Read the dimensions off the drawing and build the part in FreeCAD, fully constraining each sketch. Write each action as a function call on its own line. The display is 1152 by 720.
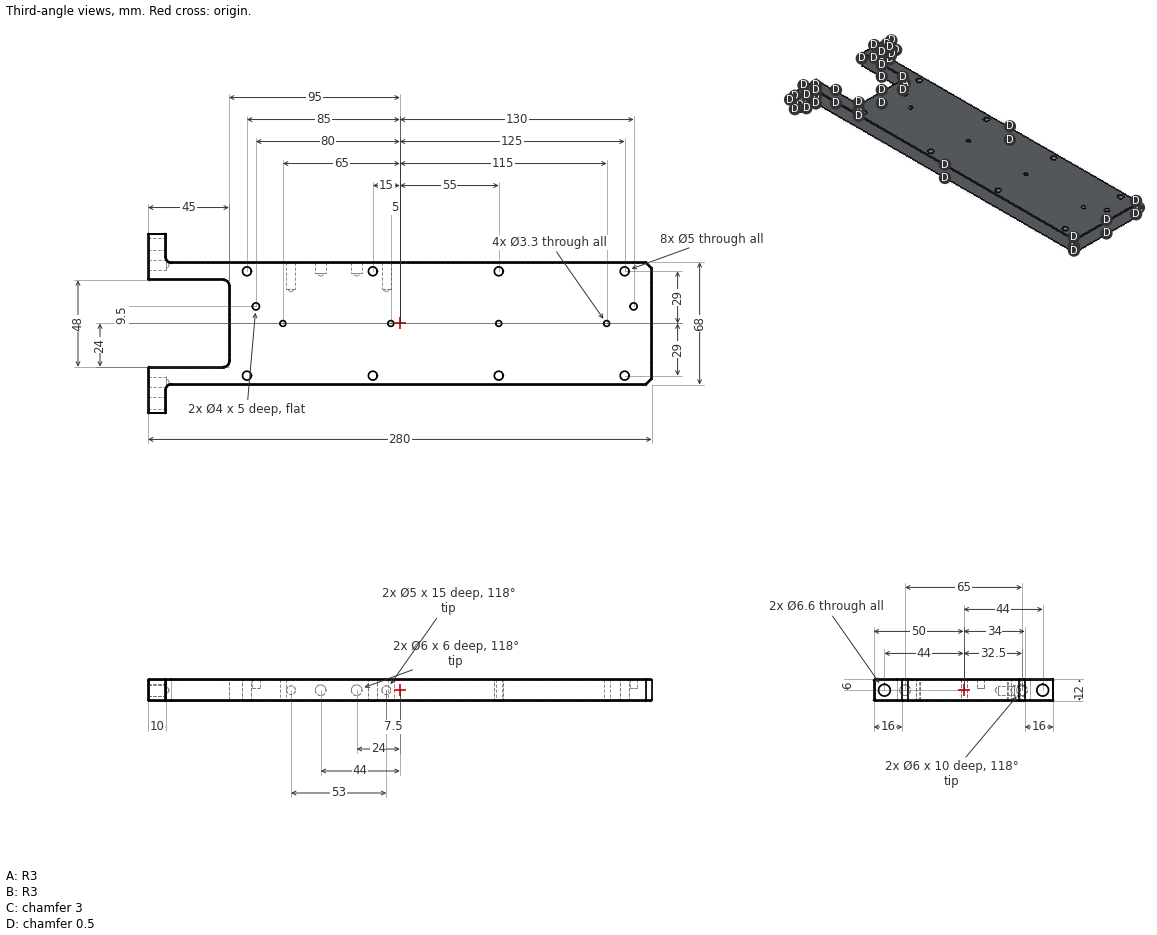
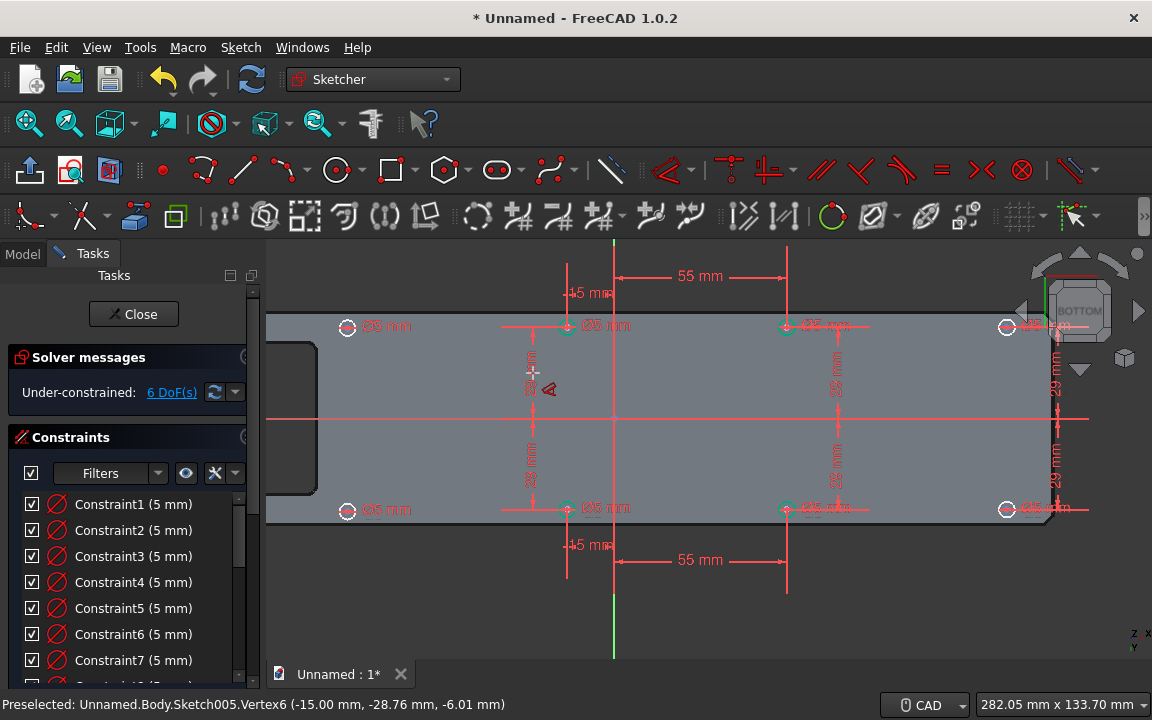
click(348, 512)
click(481, 546)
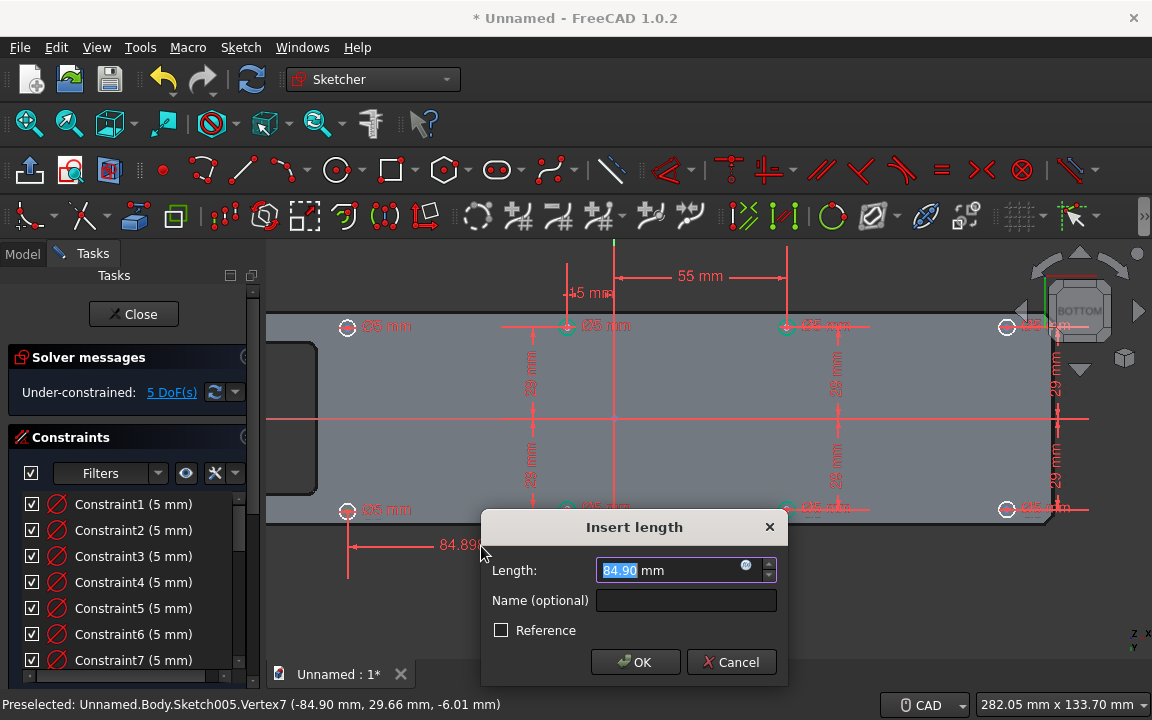
text(85)
key(Return)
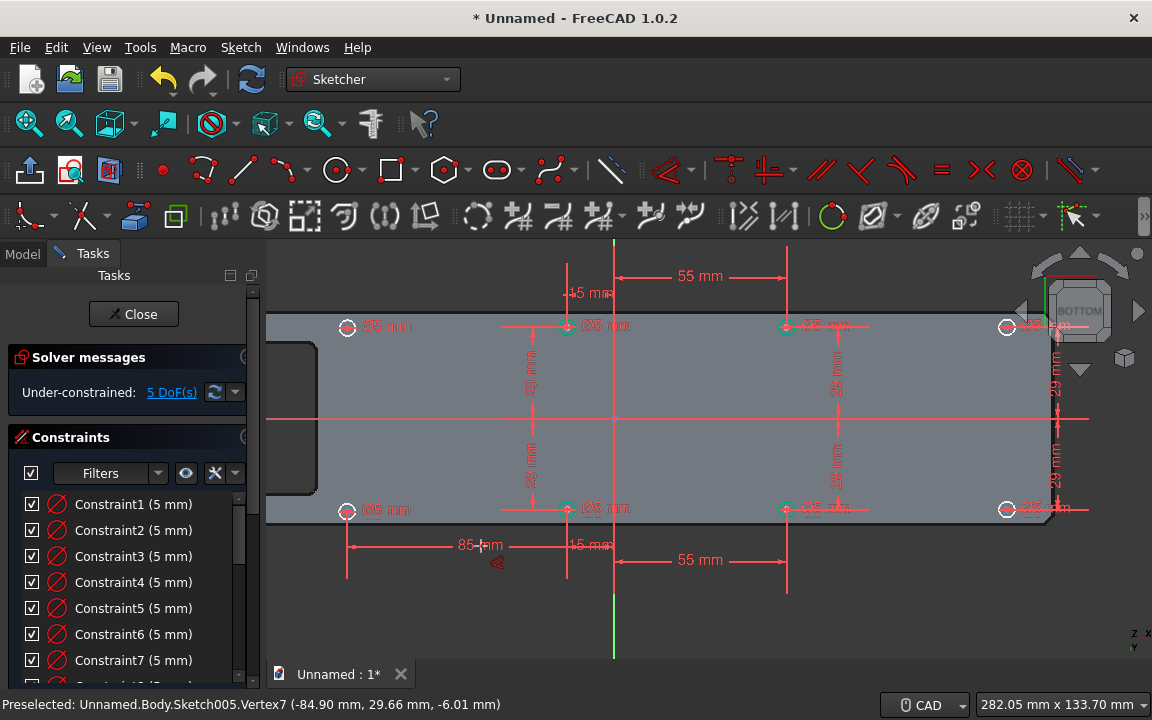
click(347, 512)
click(313, 465)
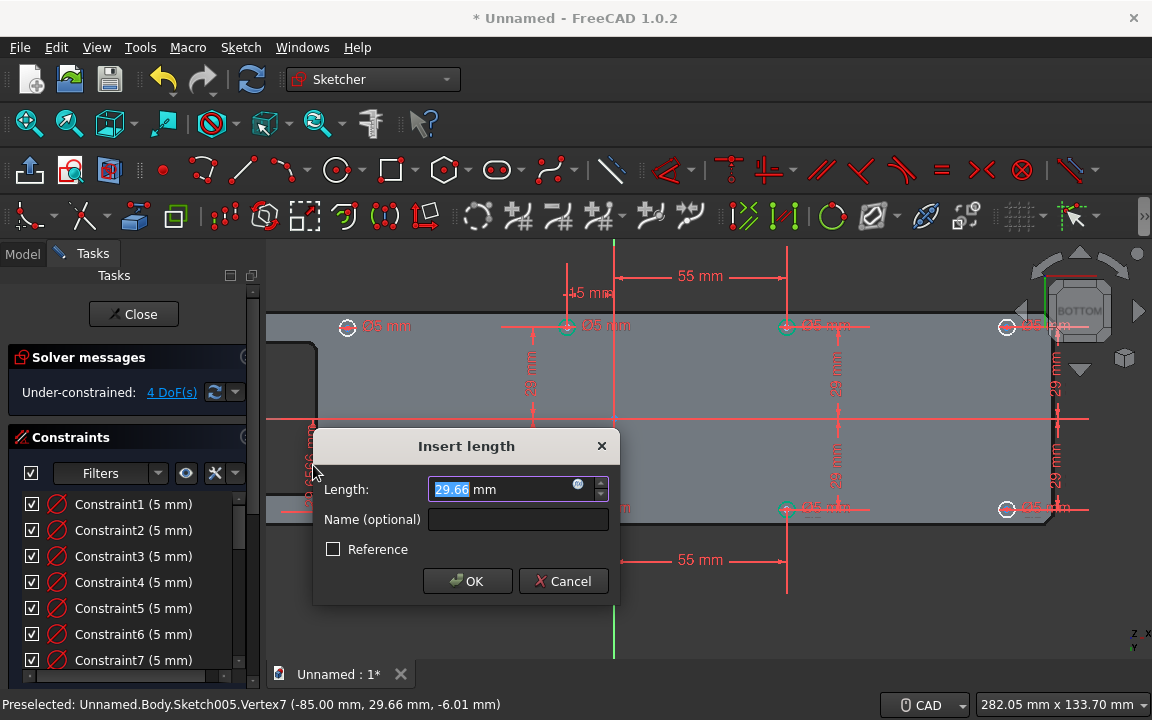
text(29)
key(Return)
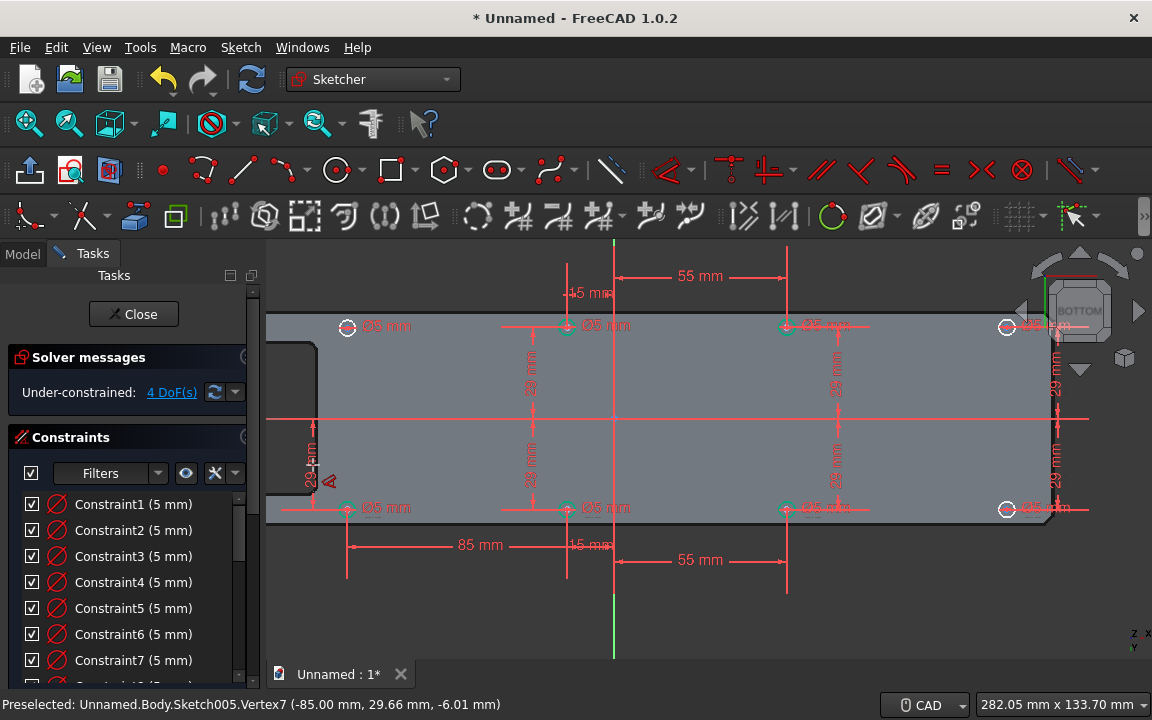
click(348, 328)
click(481, 294)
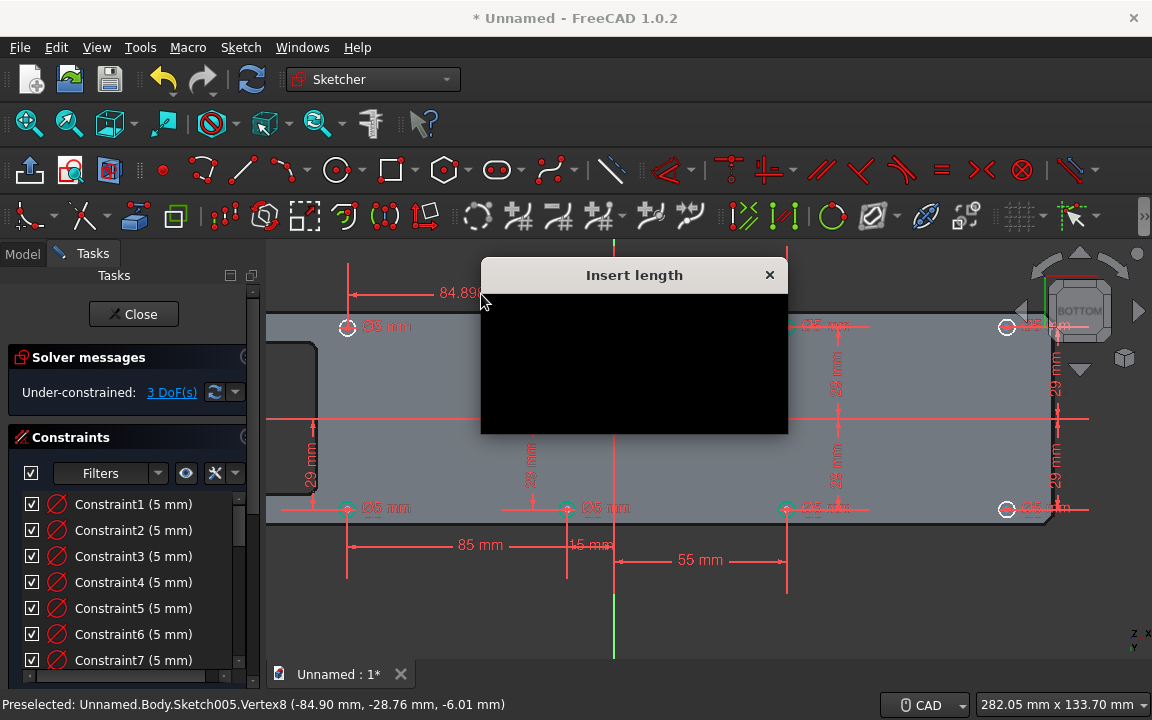
text(85)
key(Return)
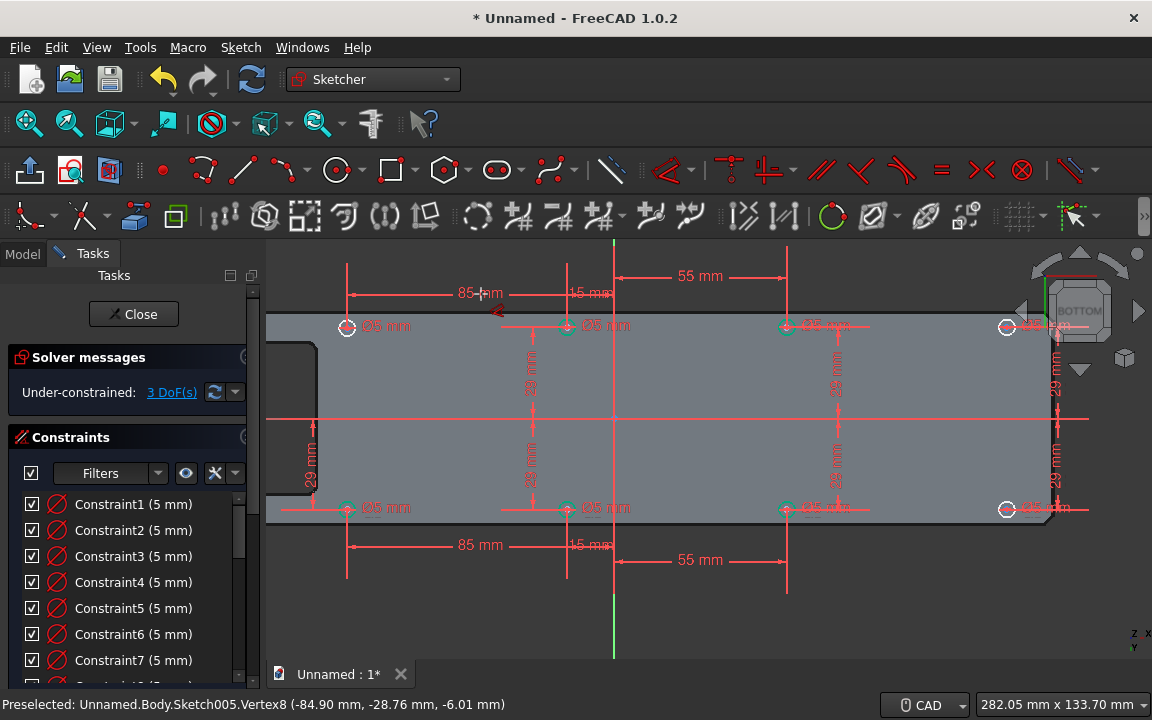
click(347, 328)
click(313, 373)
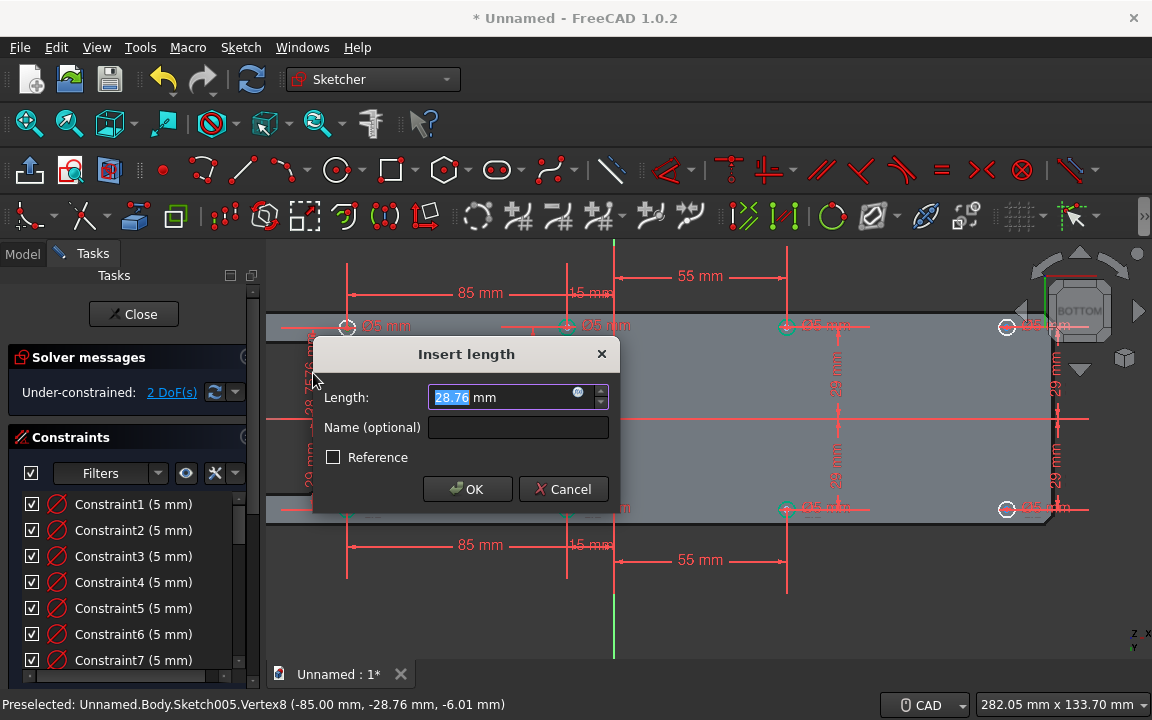
text(29)
key(Return)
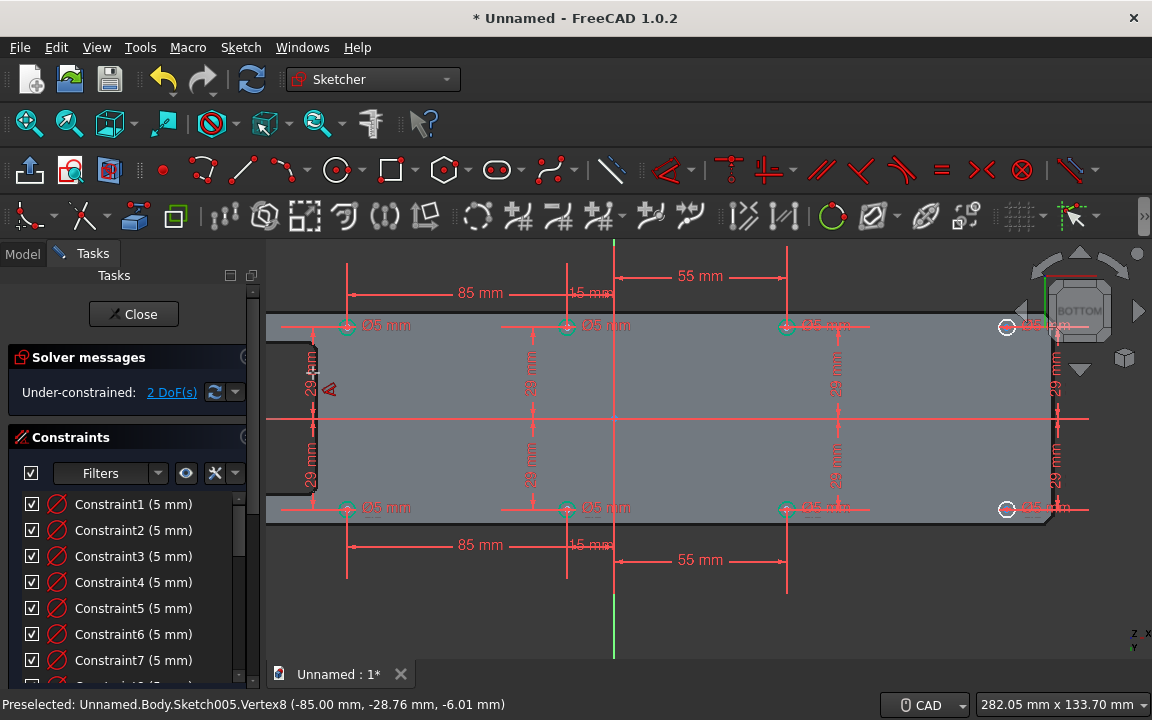
scroll(566, 511, down, 2)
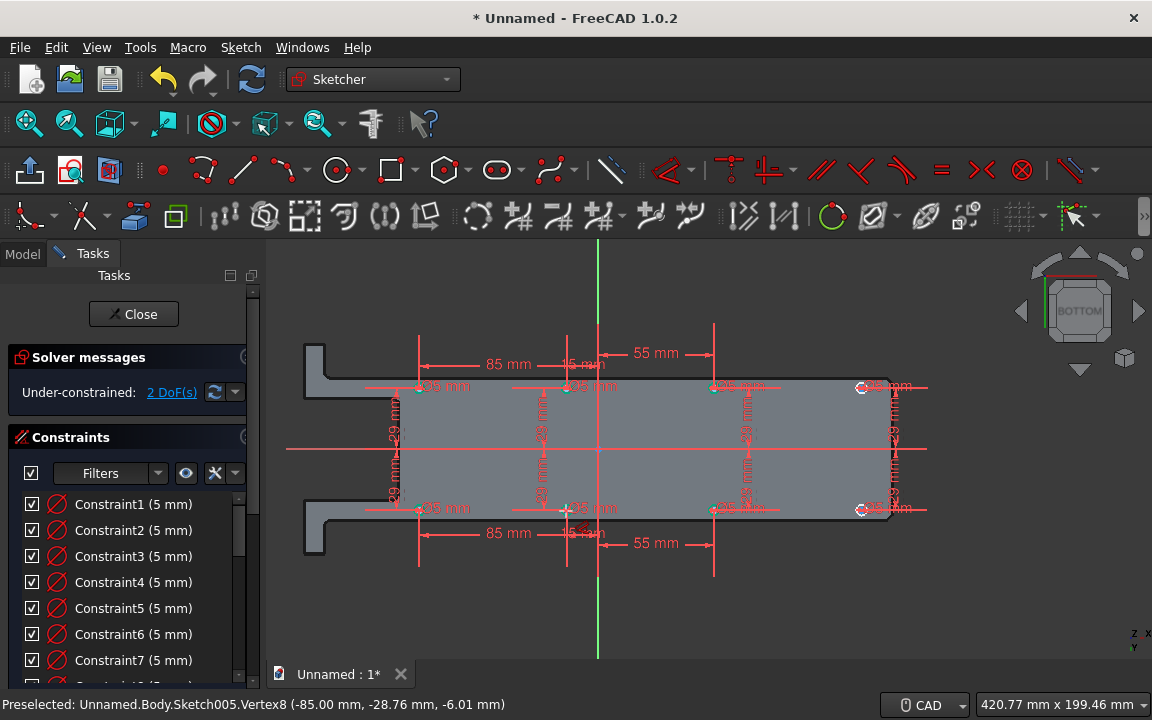
click(862, 510)
click(730, 544)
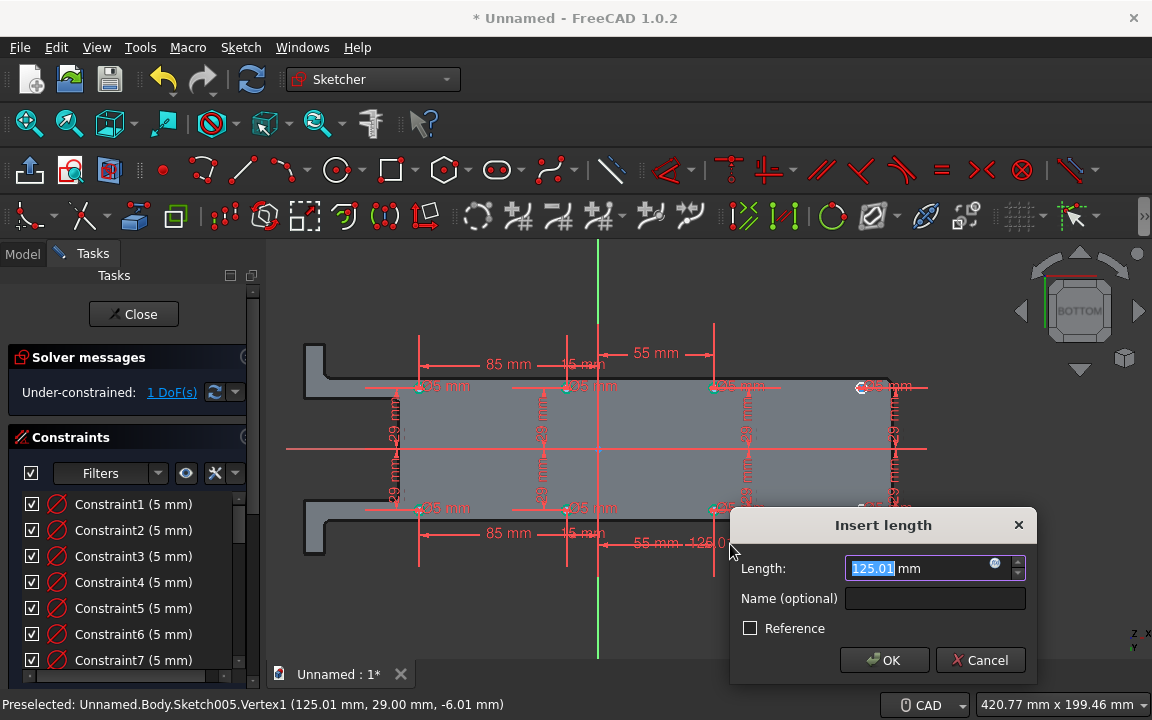
text(125)
key(Return)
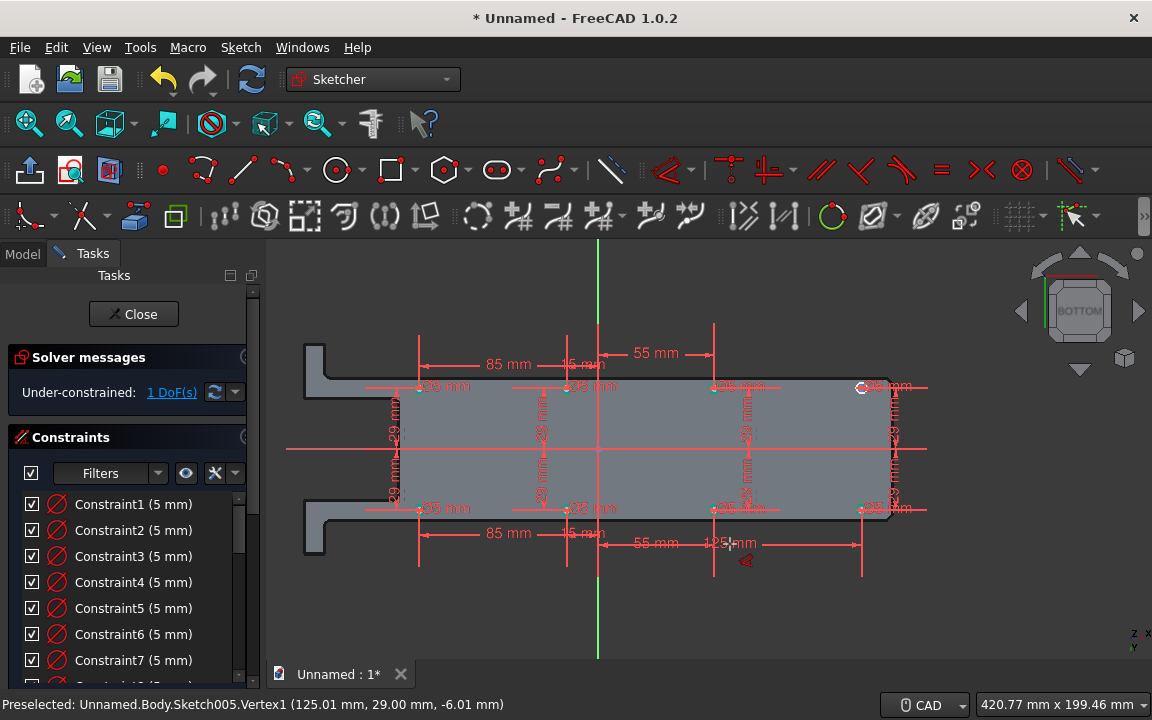
click(862, 388)
click(730, 354)